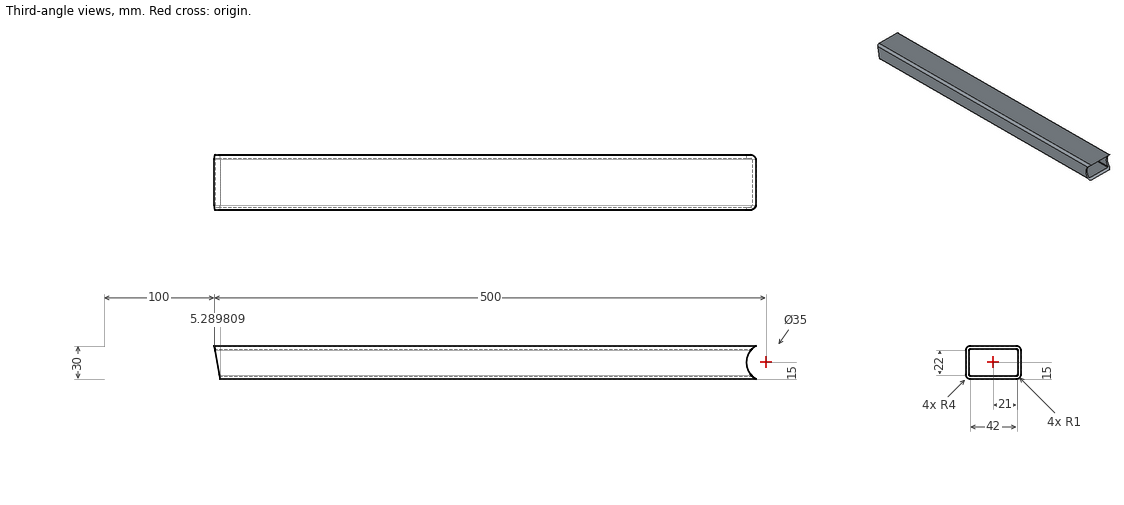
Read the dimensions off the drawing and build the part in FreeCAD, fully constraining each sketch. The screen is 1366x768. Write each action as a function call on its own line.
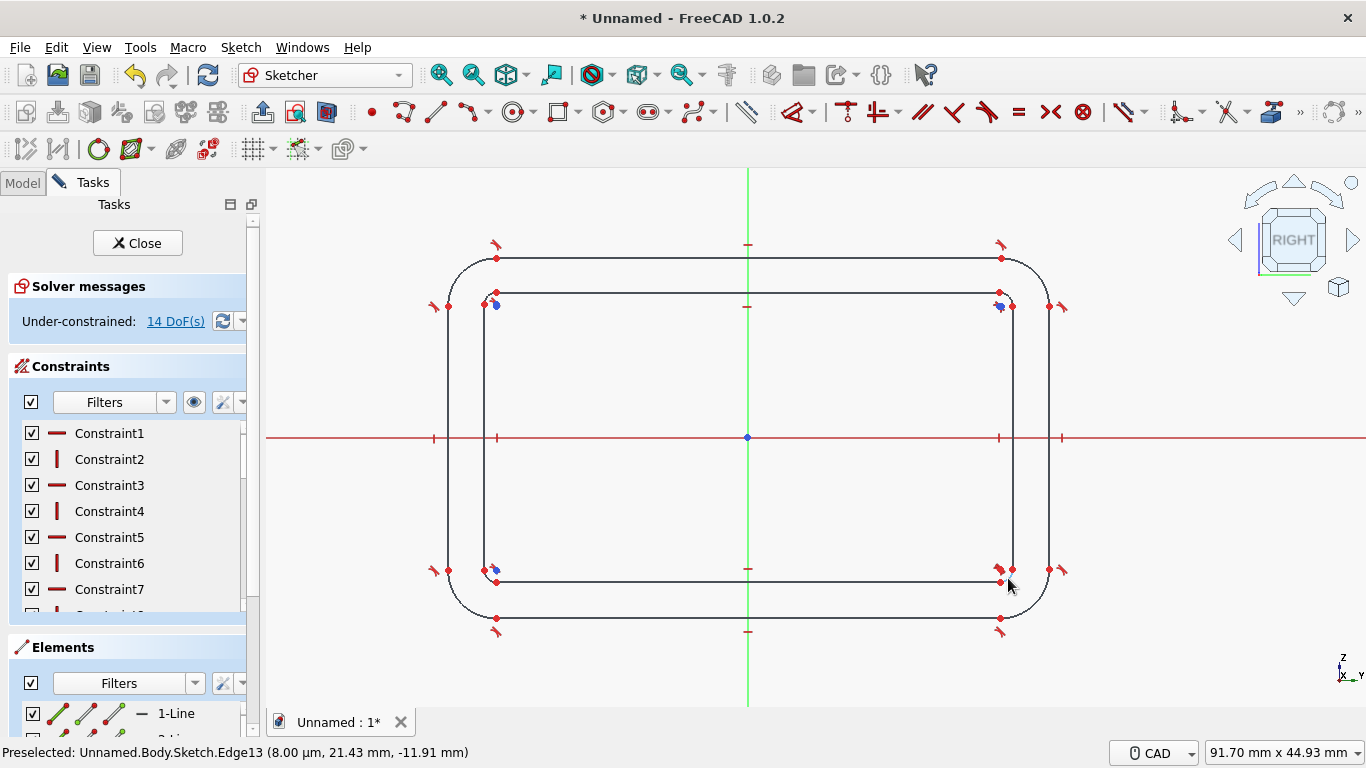
click(1044, 285)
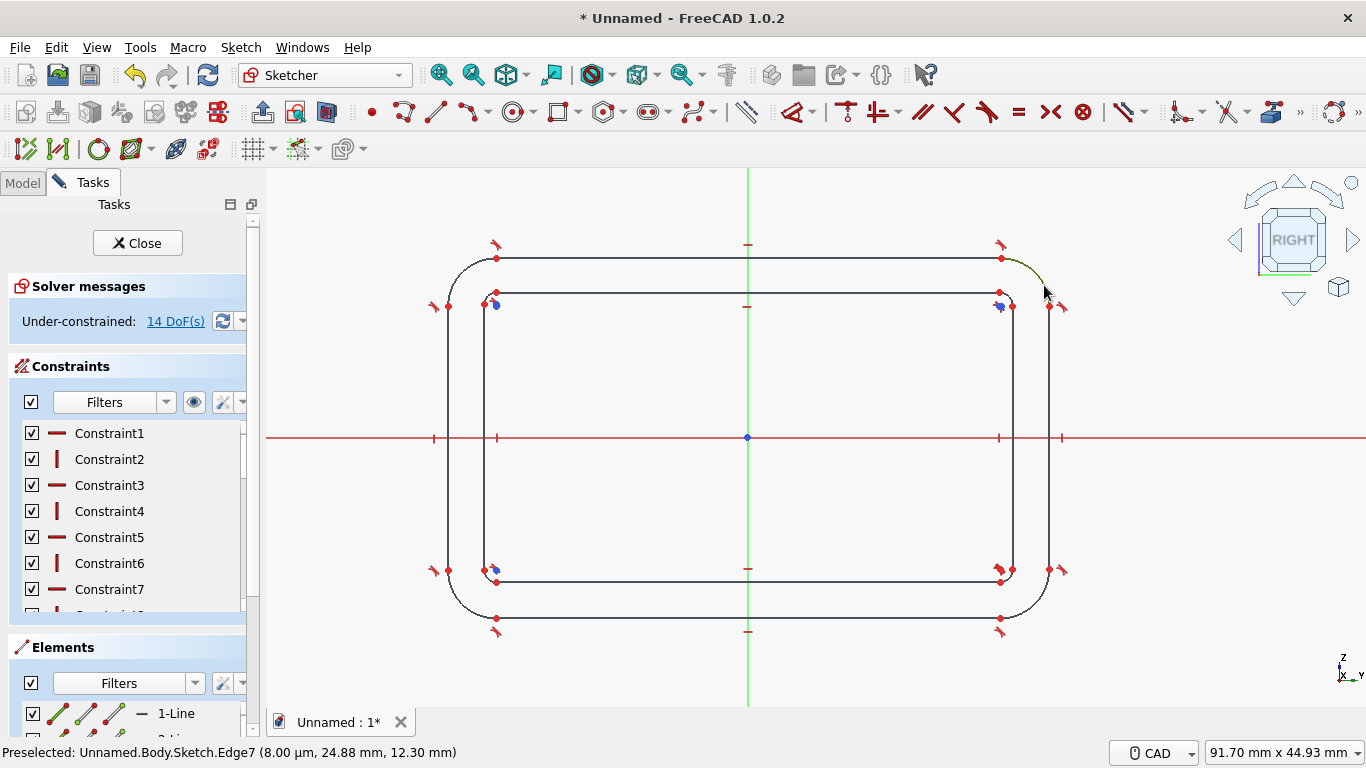
scroll(1009, 297, up, 2)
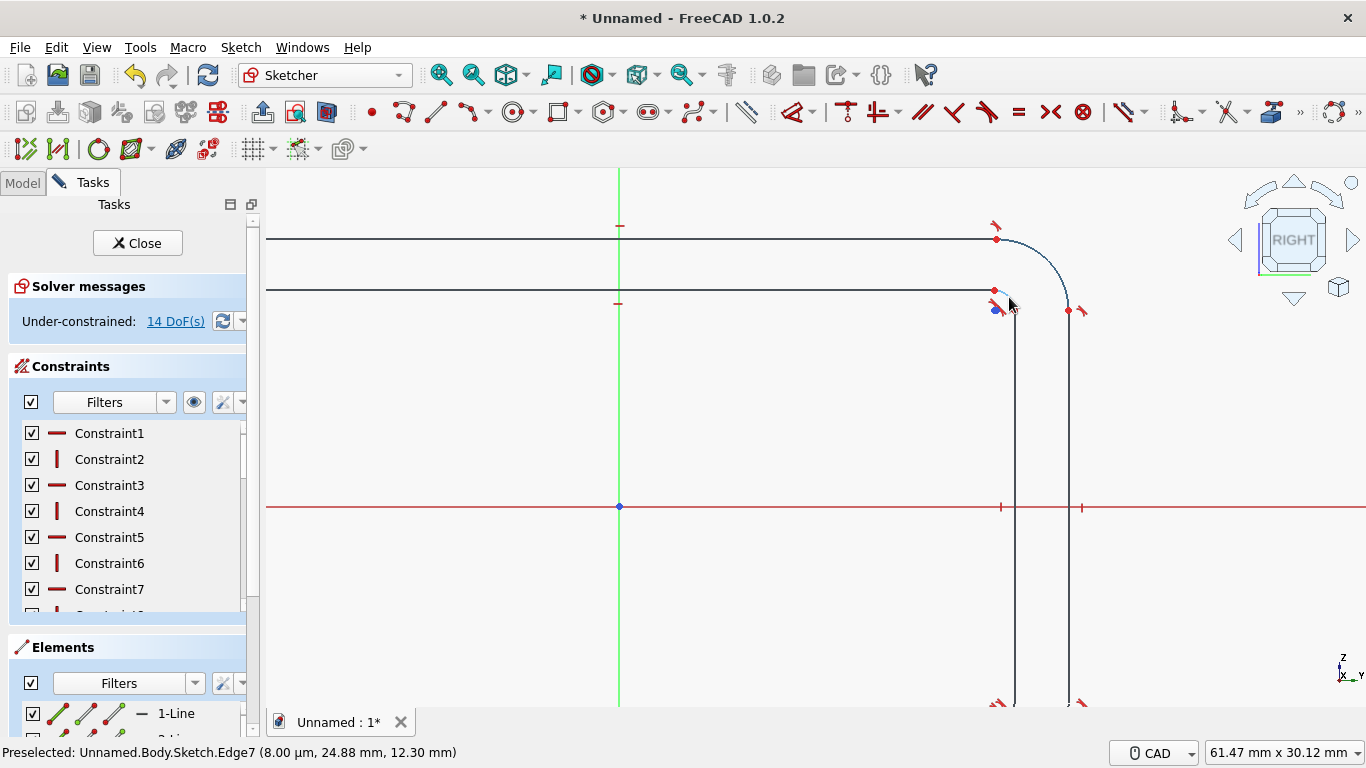
click(1009, 296)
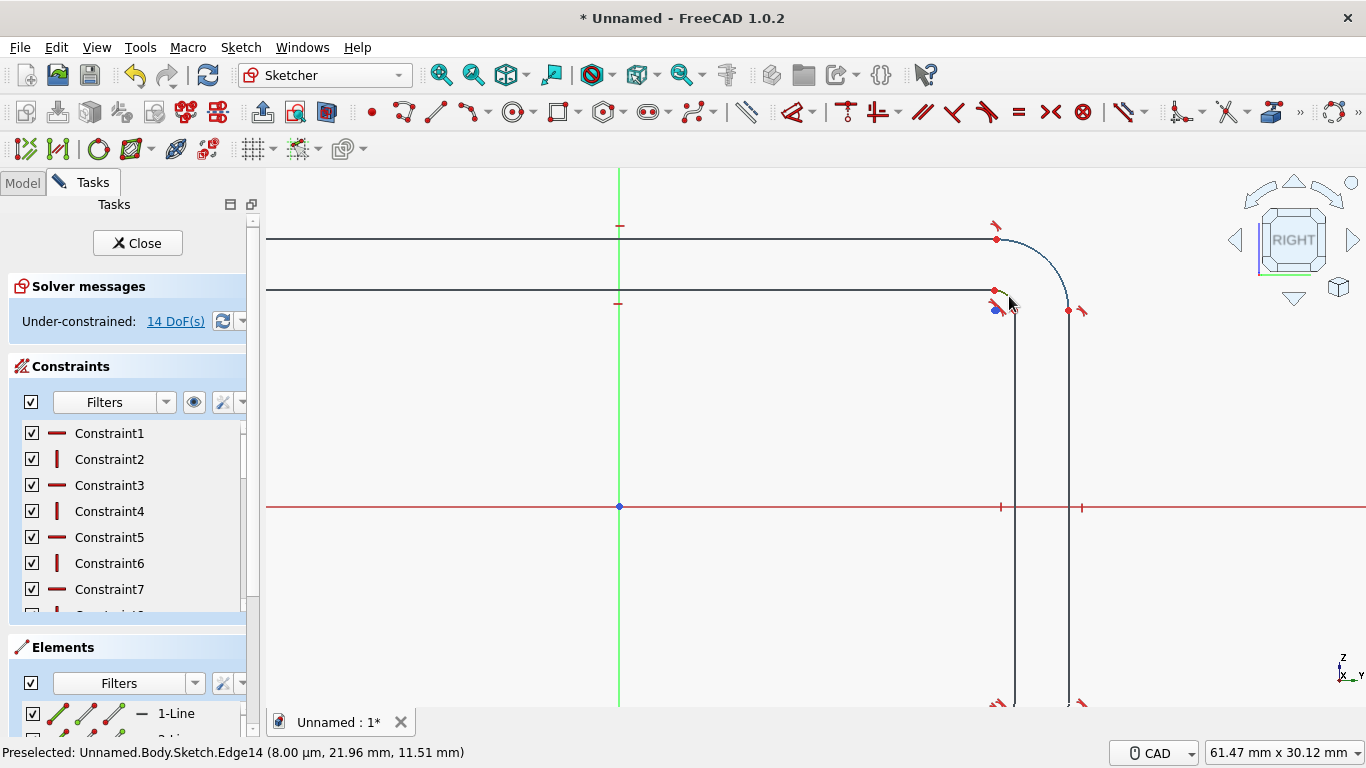
key(c)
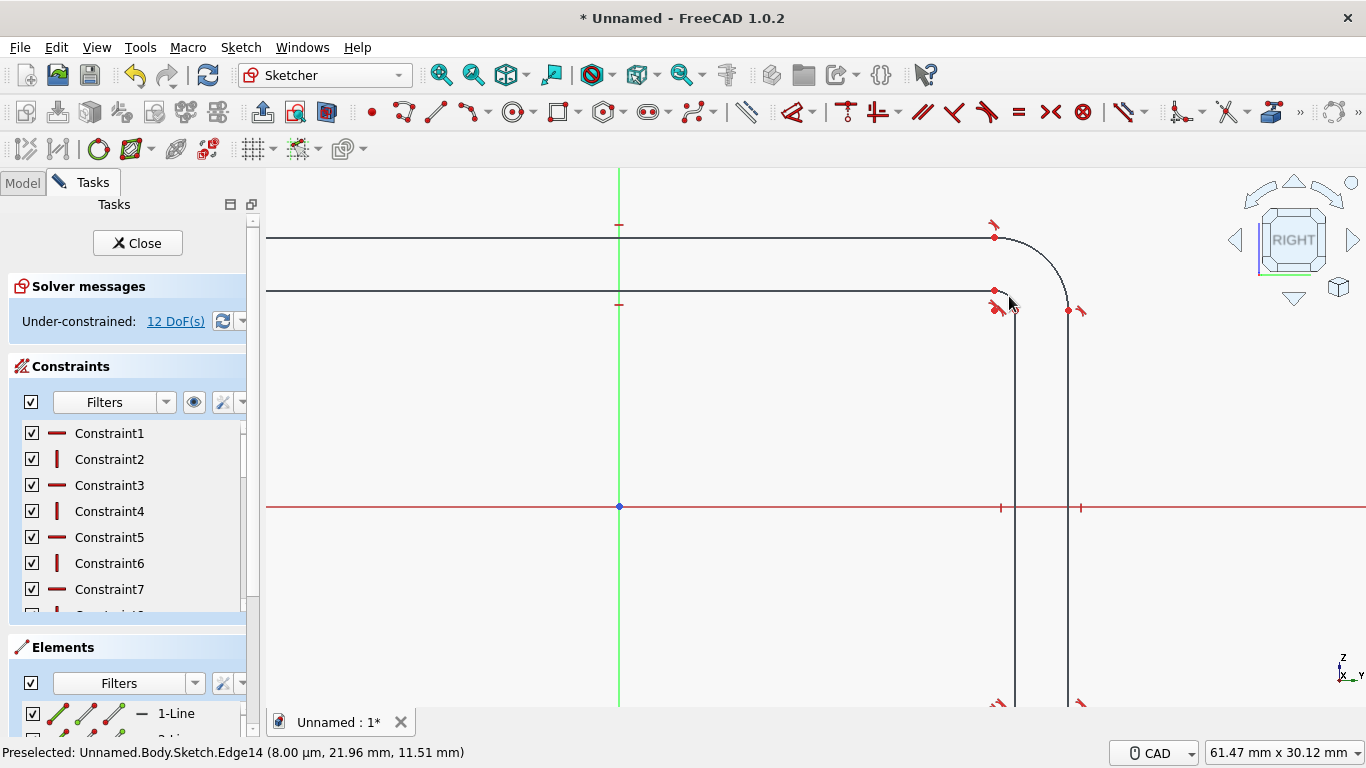
scroll(1009, 297, down, 2)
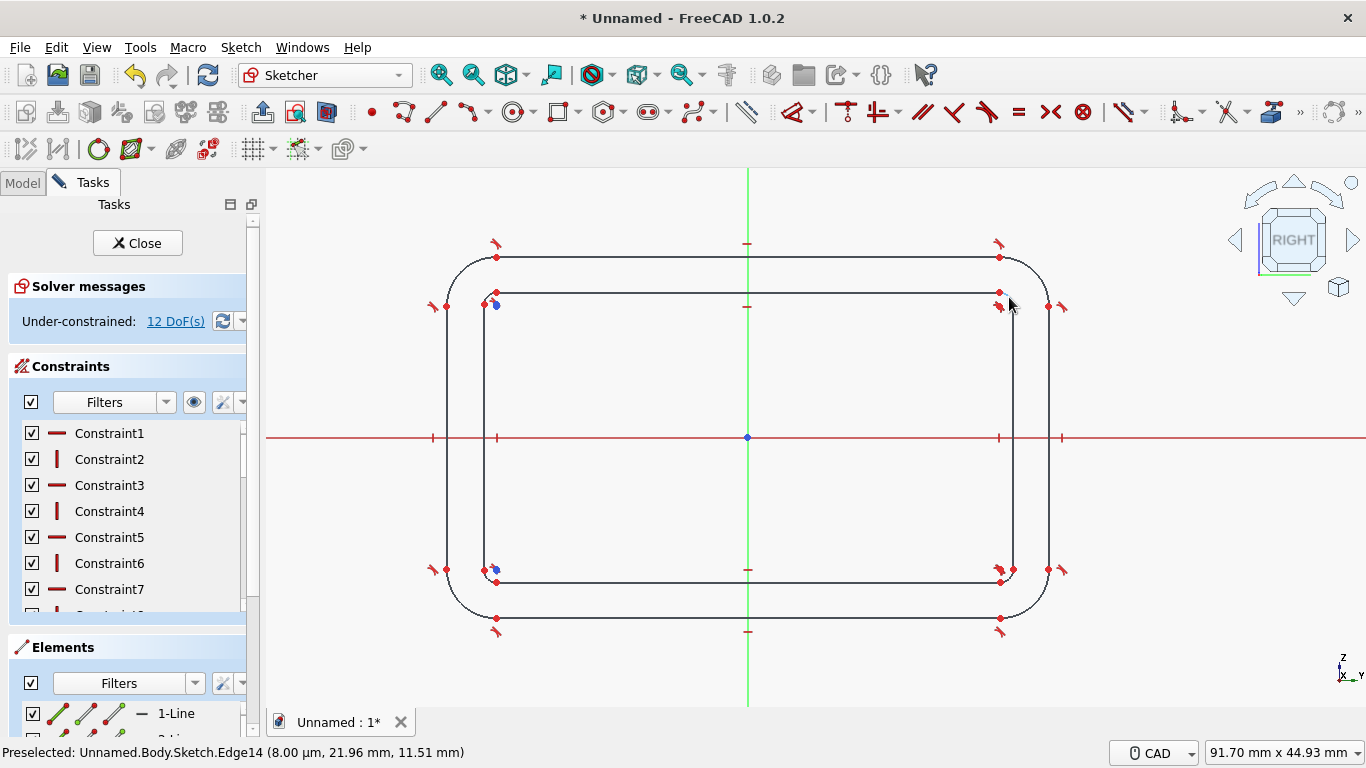
click(474, 263)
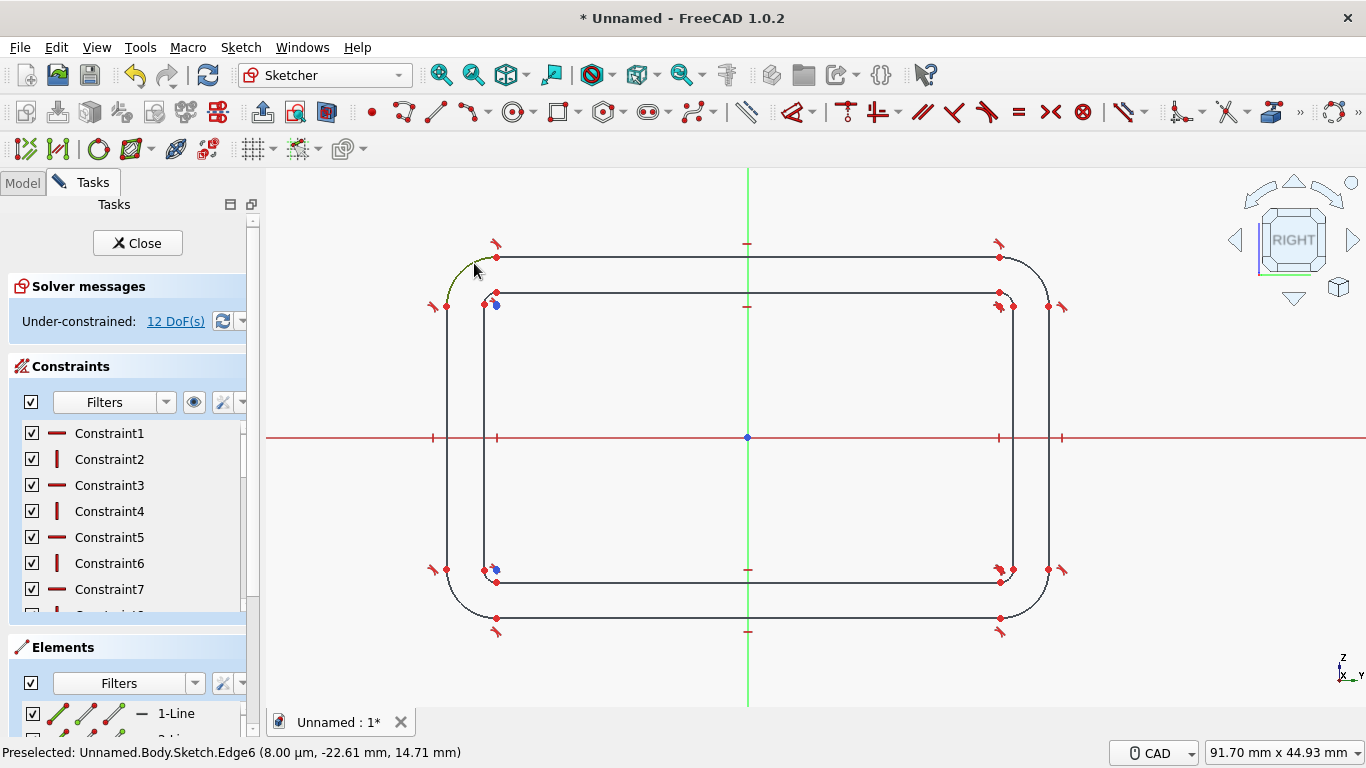
scroll(488, 296, up, 3)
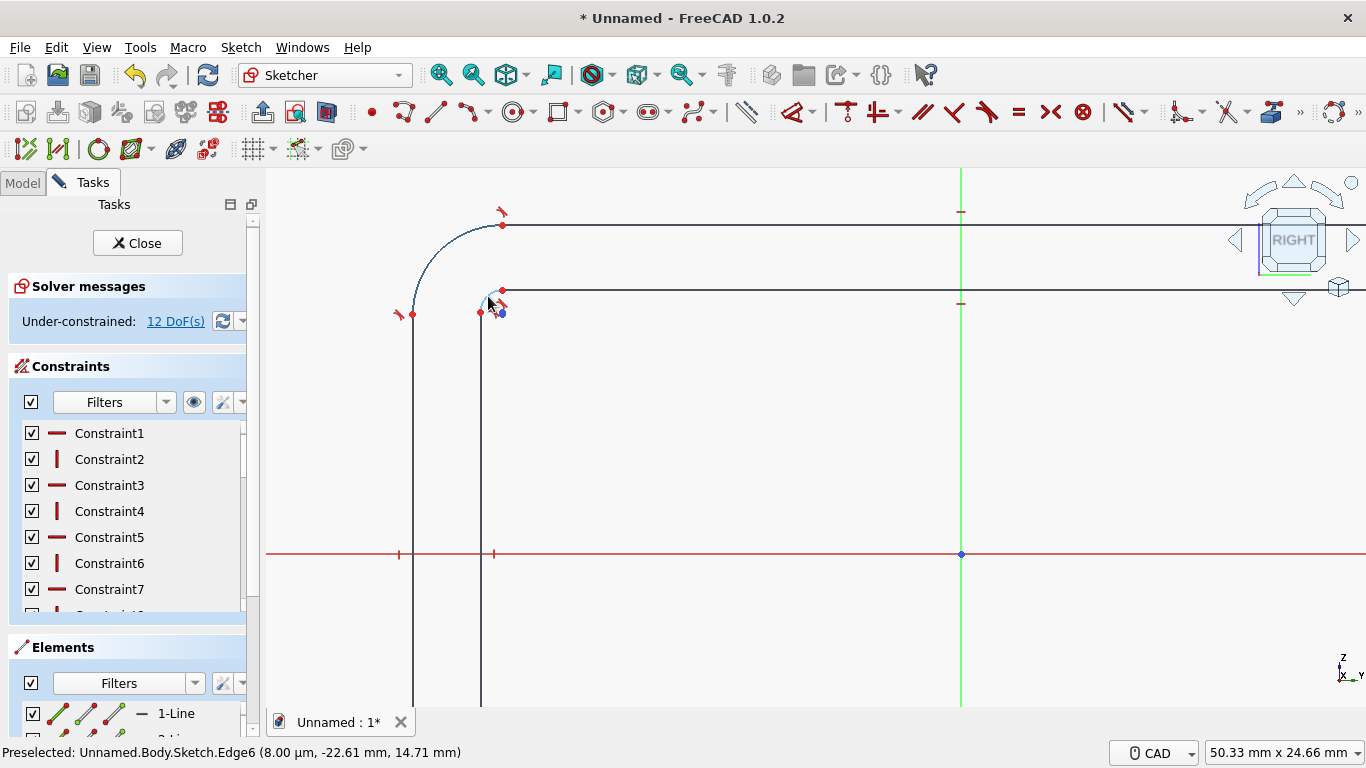
click(487, 297)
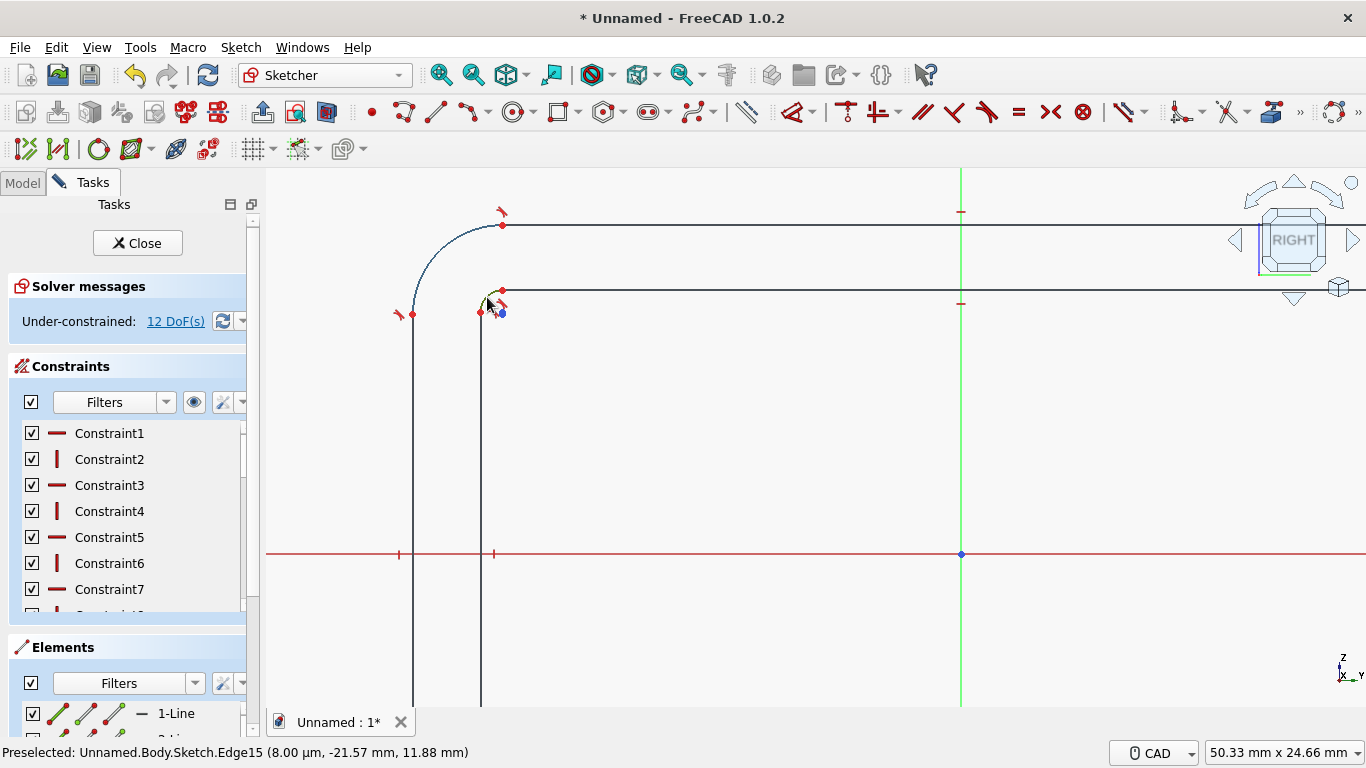
key(c)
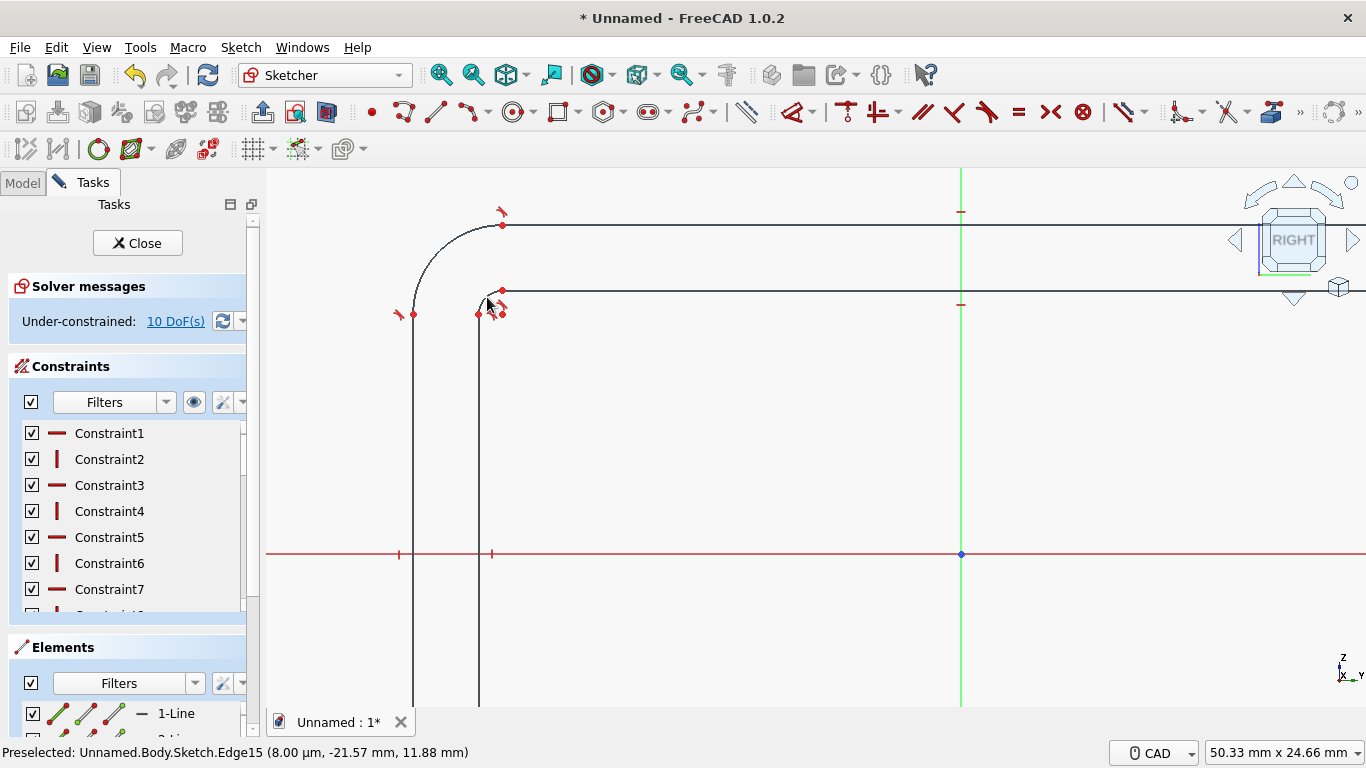
scroll(487, 296, down, 3)